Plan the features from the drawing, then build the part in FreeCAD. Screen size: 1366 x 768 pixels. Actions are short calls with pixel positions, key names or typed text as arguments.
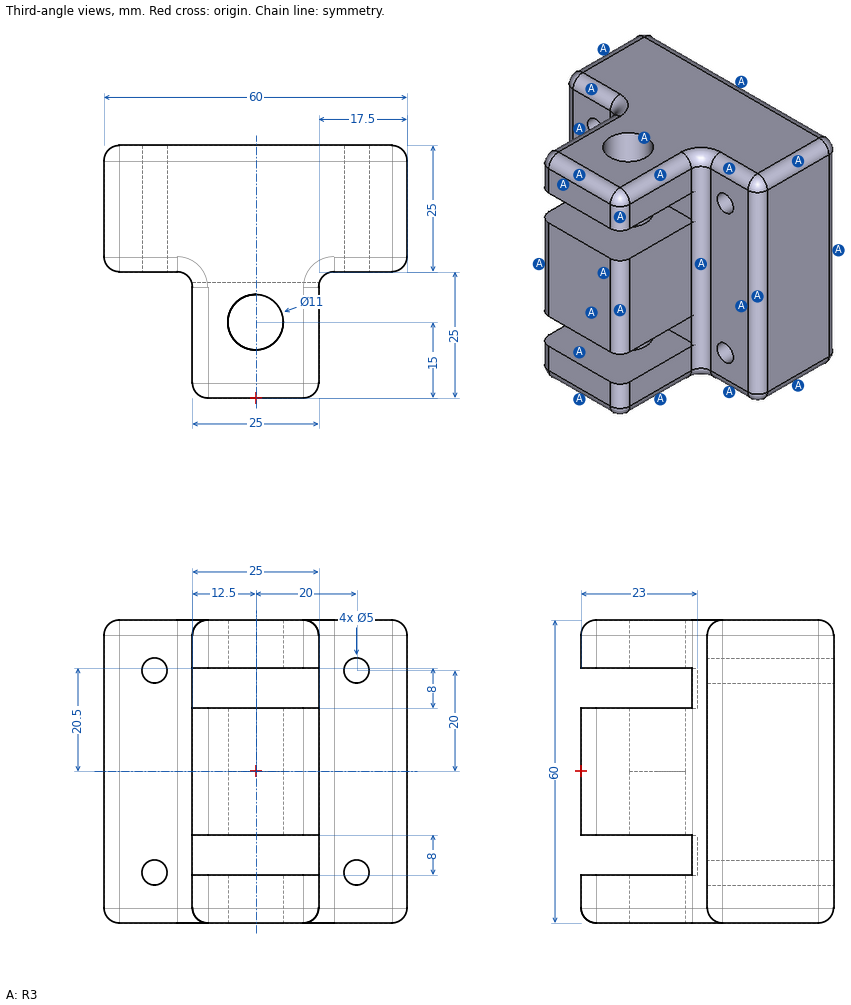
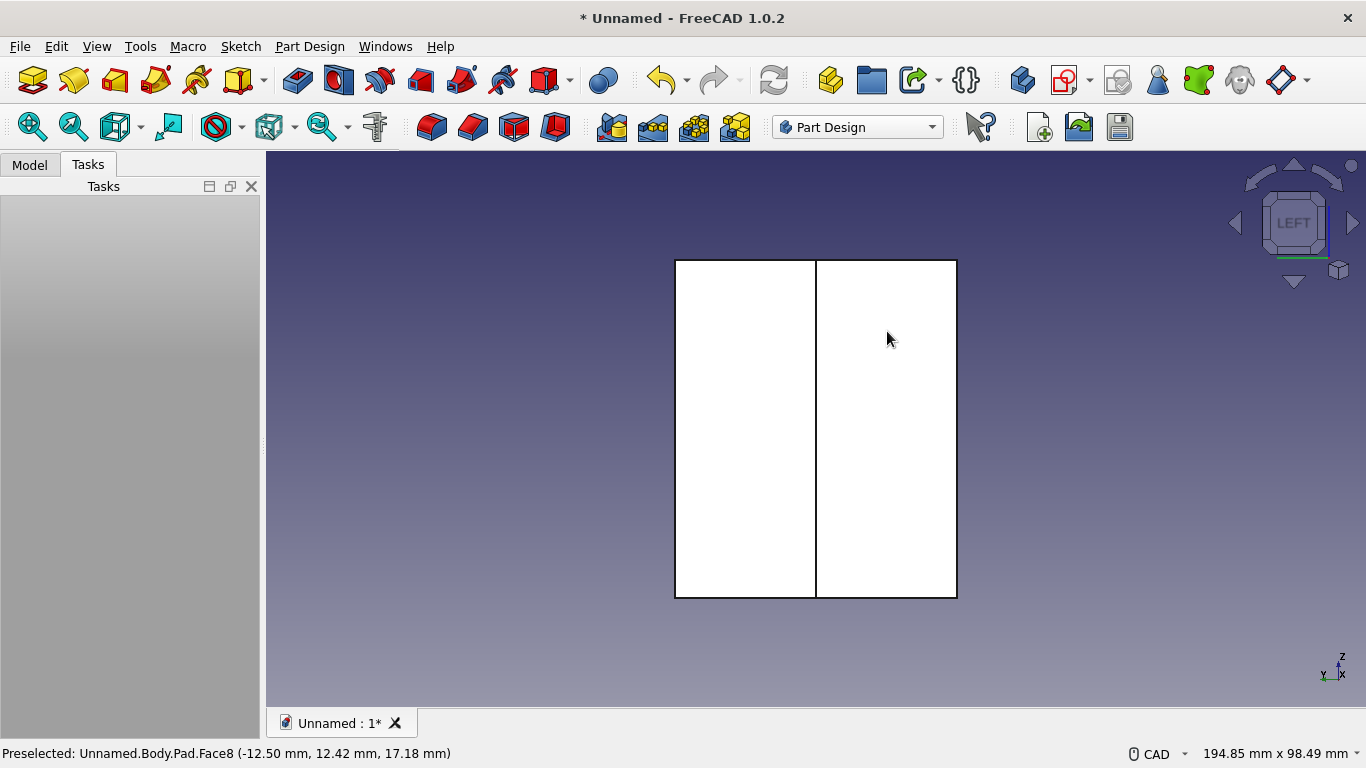
click(432, 128)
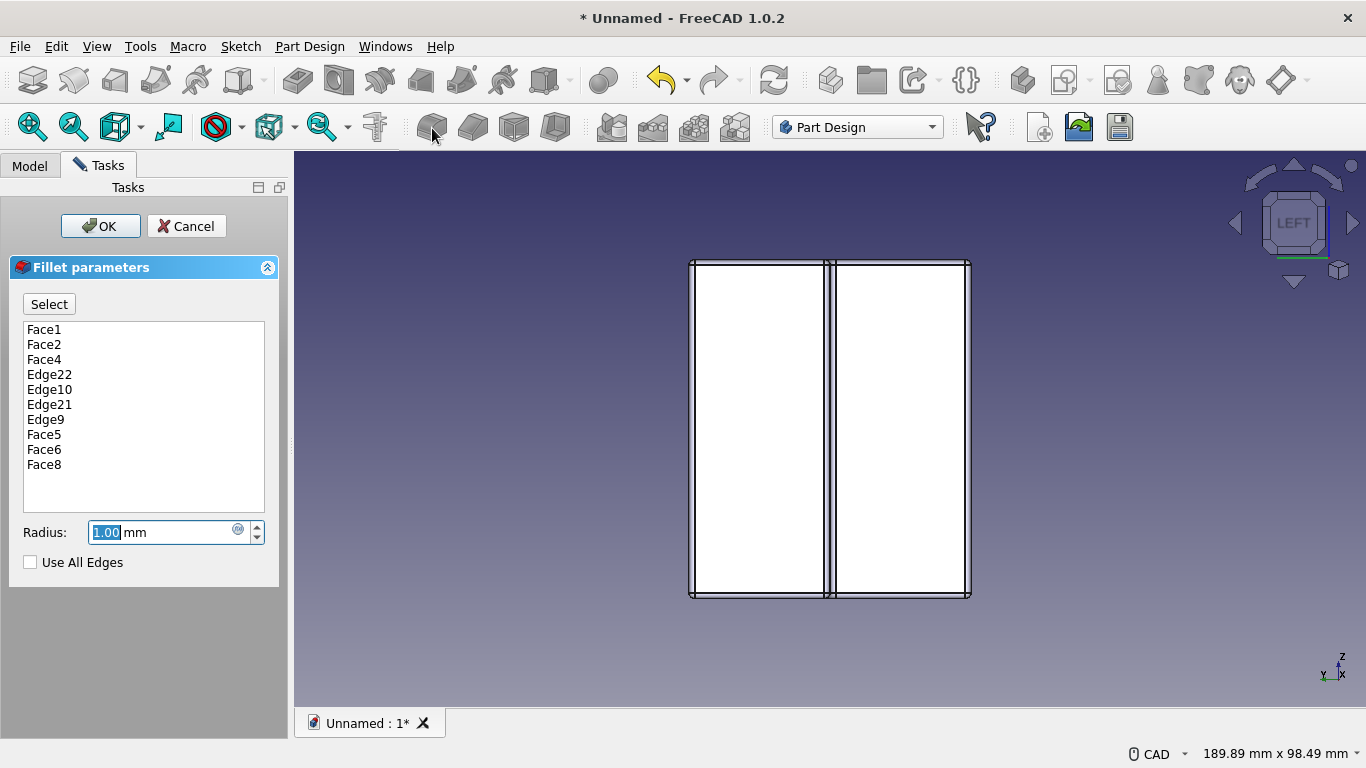
text(3)
key(Tab)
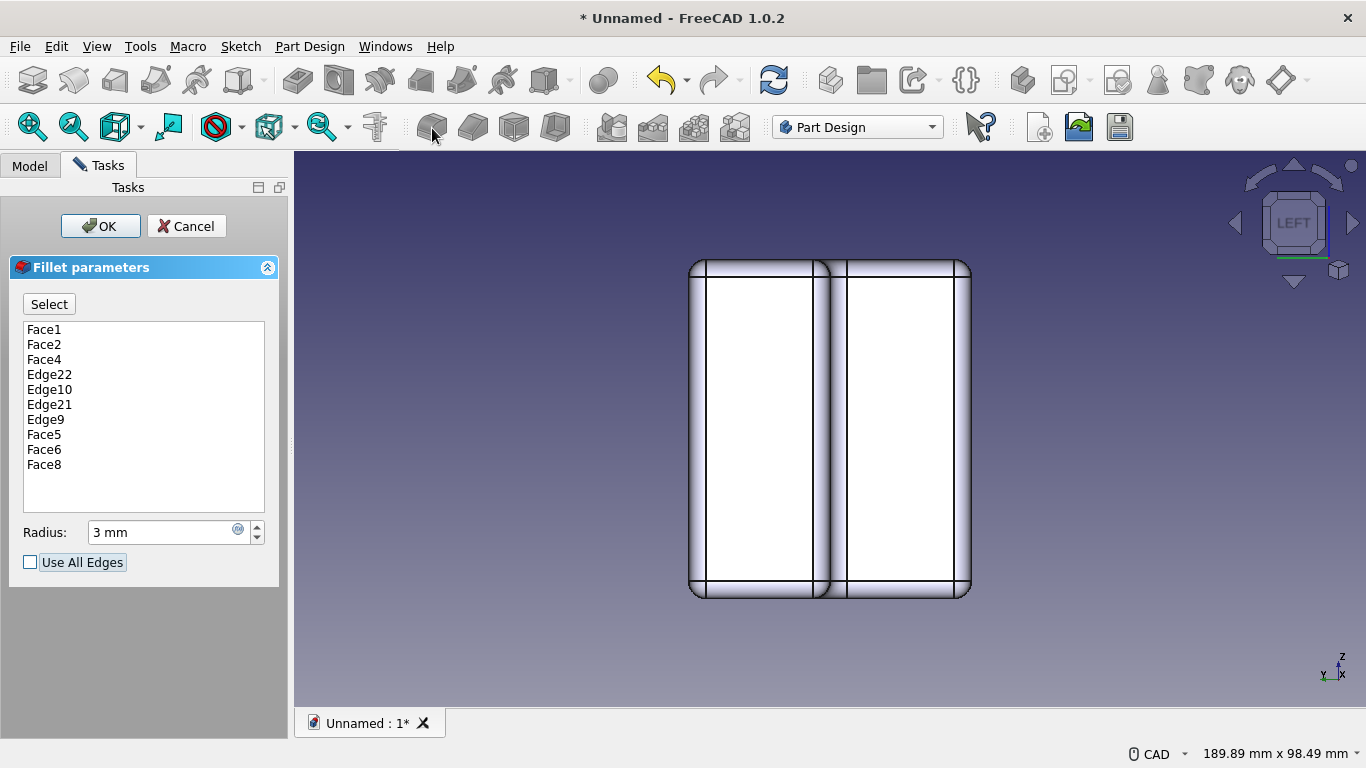
click(101, 226)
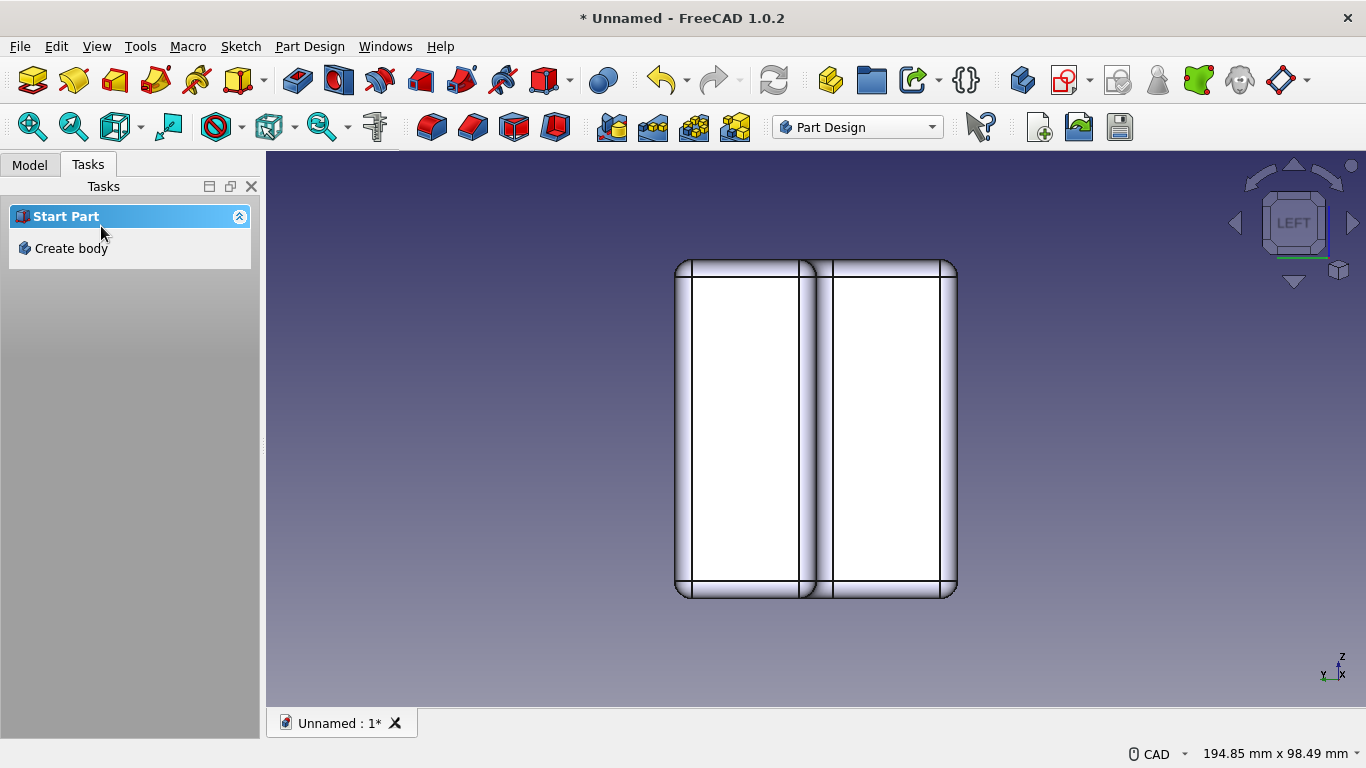
click(1064, 80)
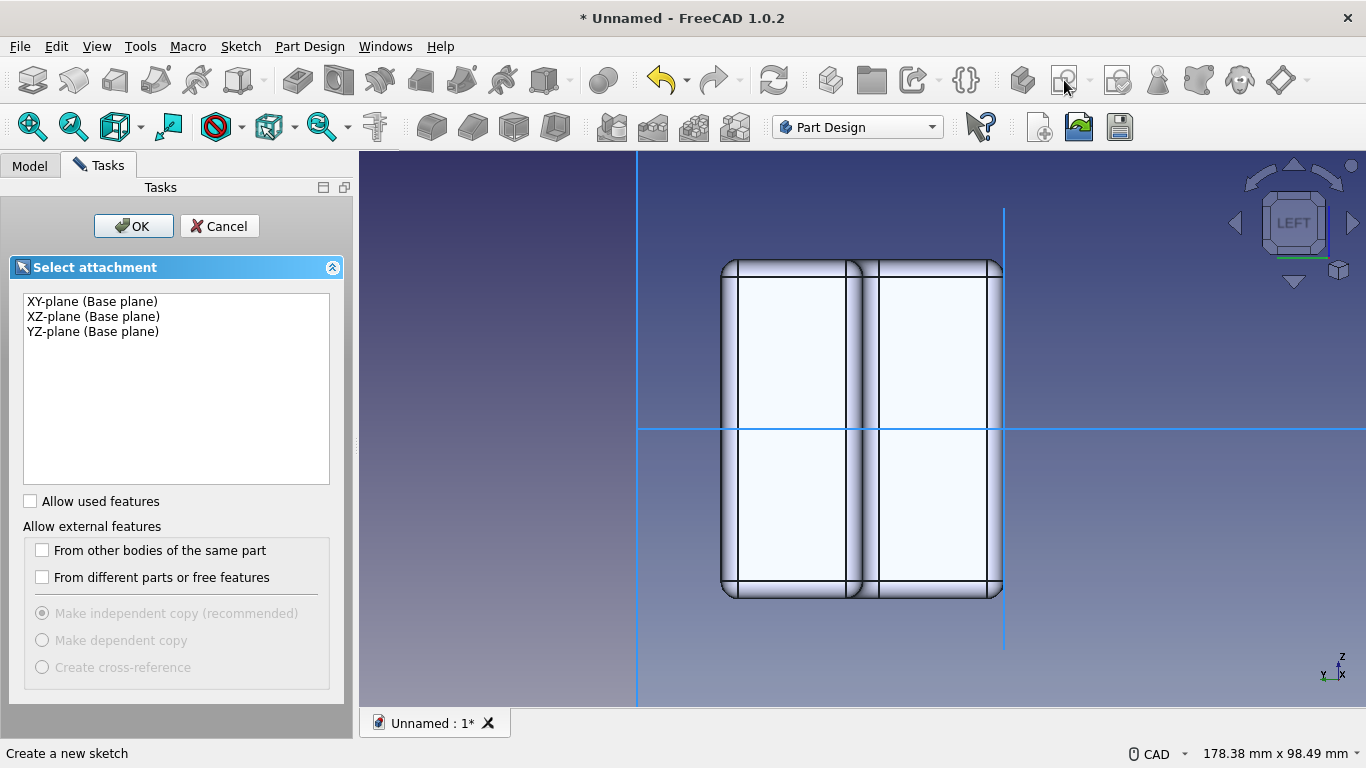
click(84, 316)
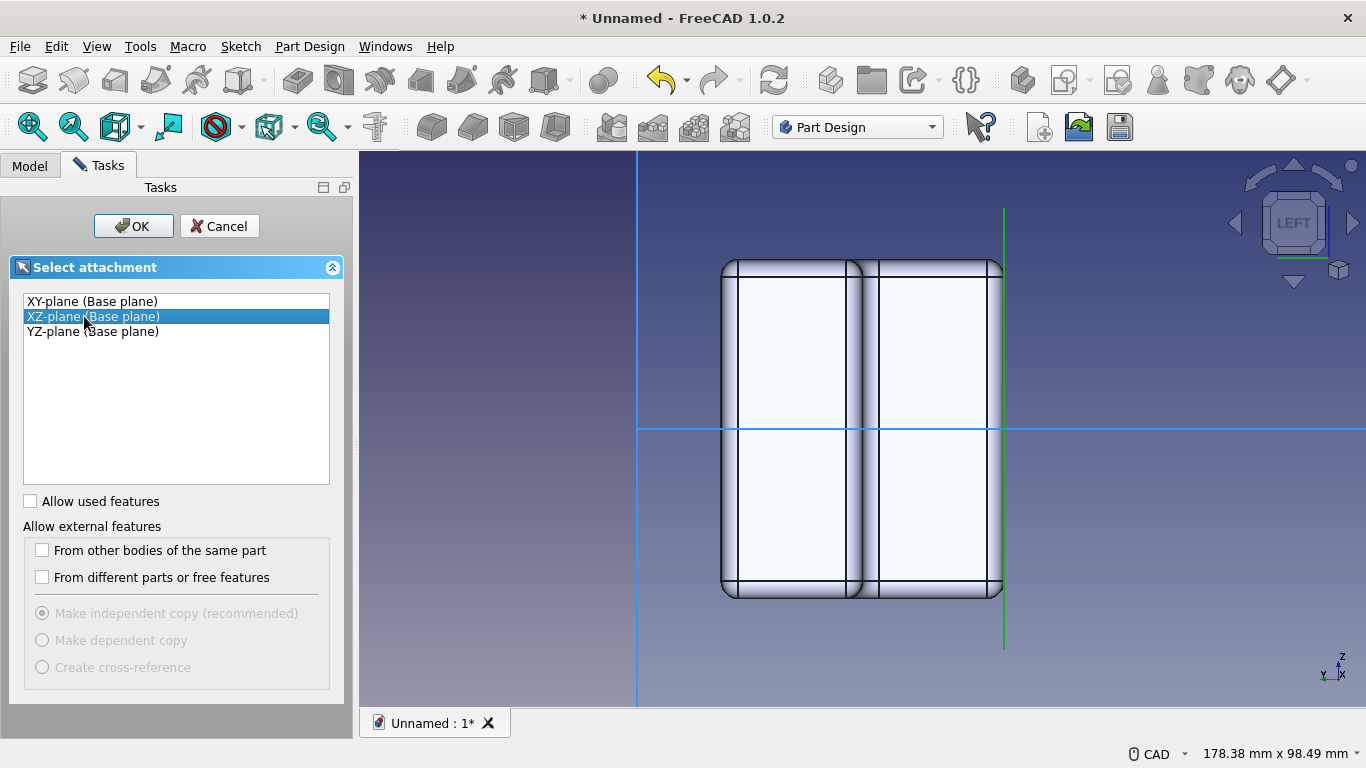
click(134, 226)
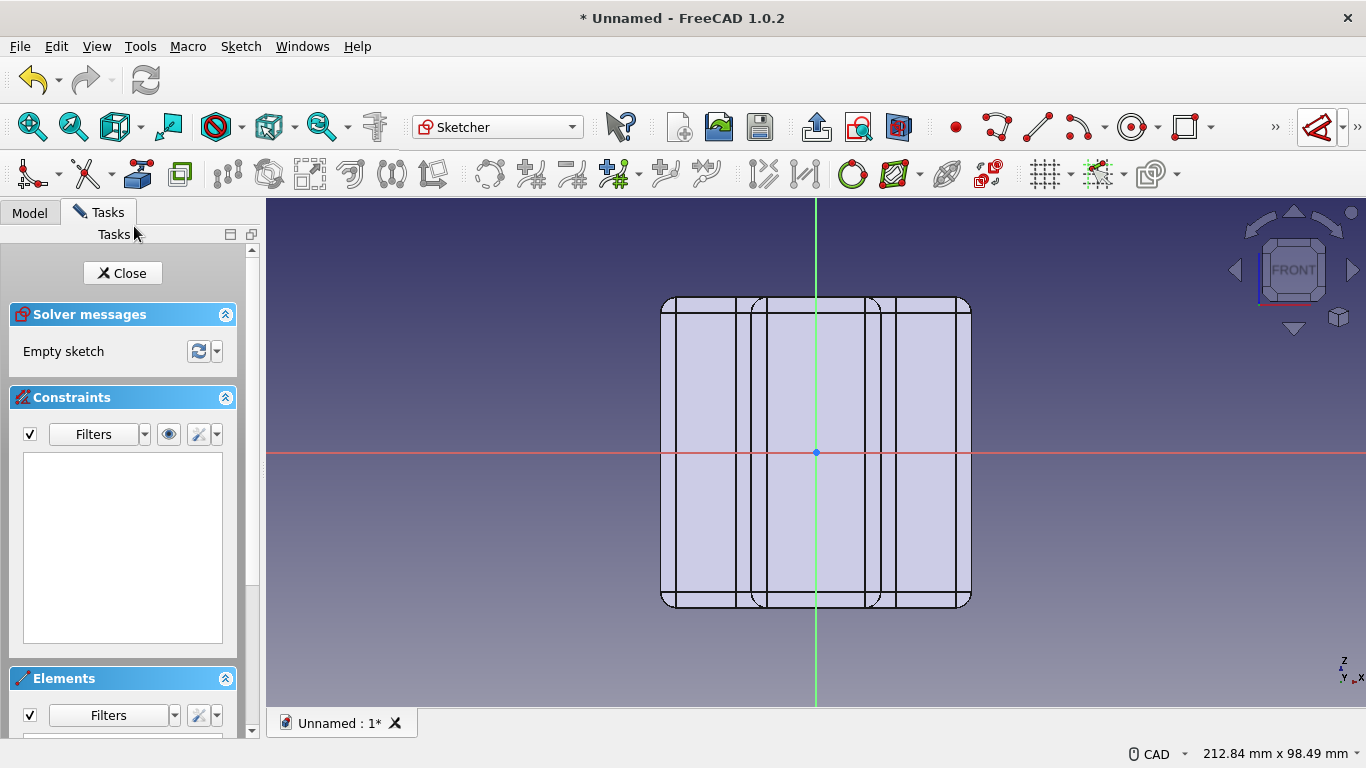
scroll(955, 453, up, 2)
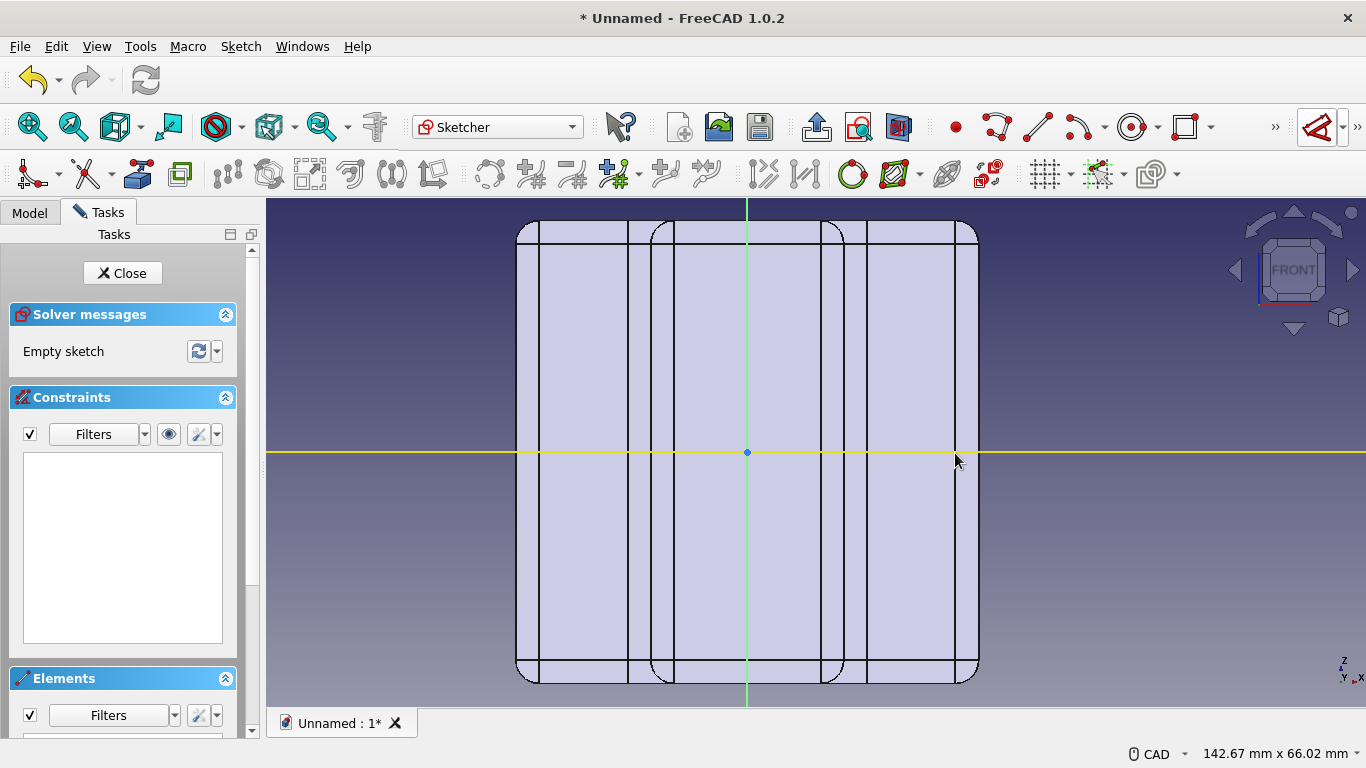
key(g)
key(r)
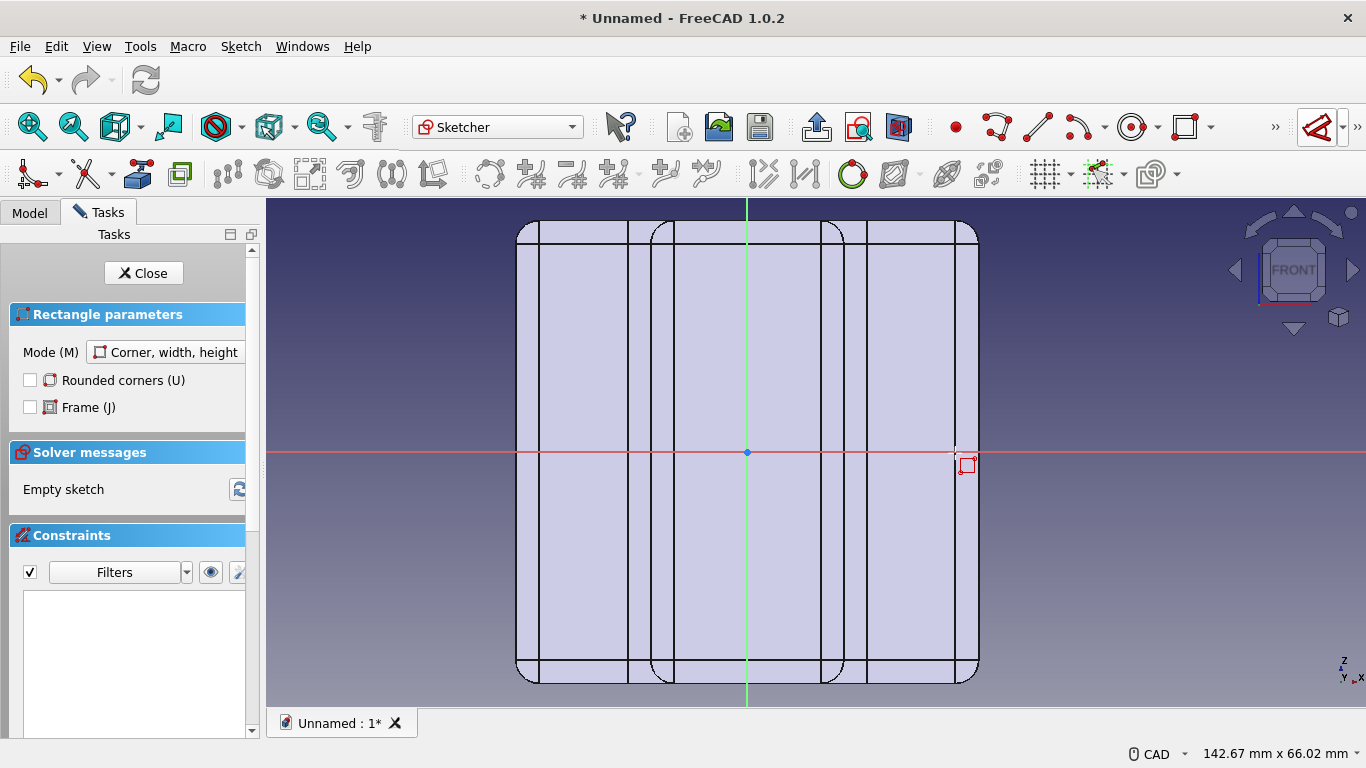
click(651, 294)
move(844, 356)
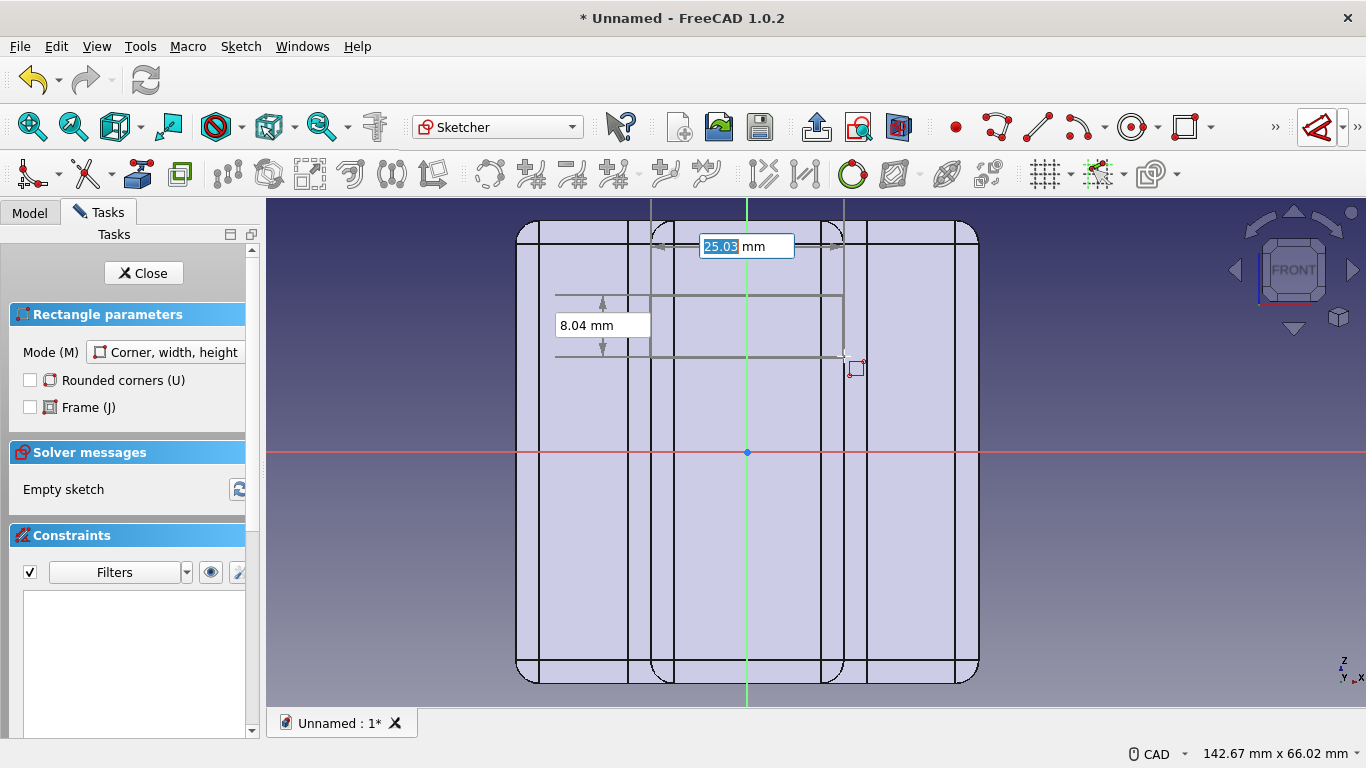
text(25)
key(Tab)
text(8)
key(Return)